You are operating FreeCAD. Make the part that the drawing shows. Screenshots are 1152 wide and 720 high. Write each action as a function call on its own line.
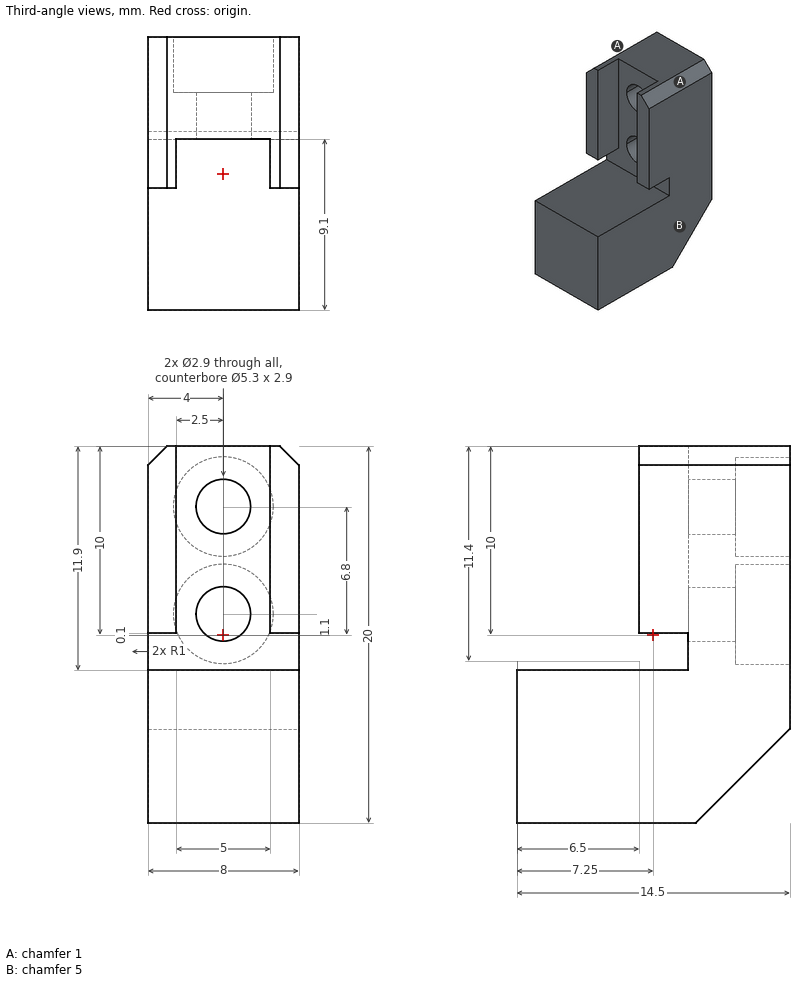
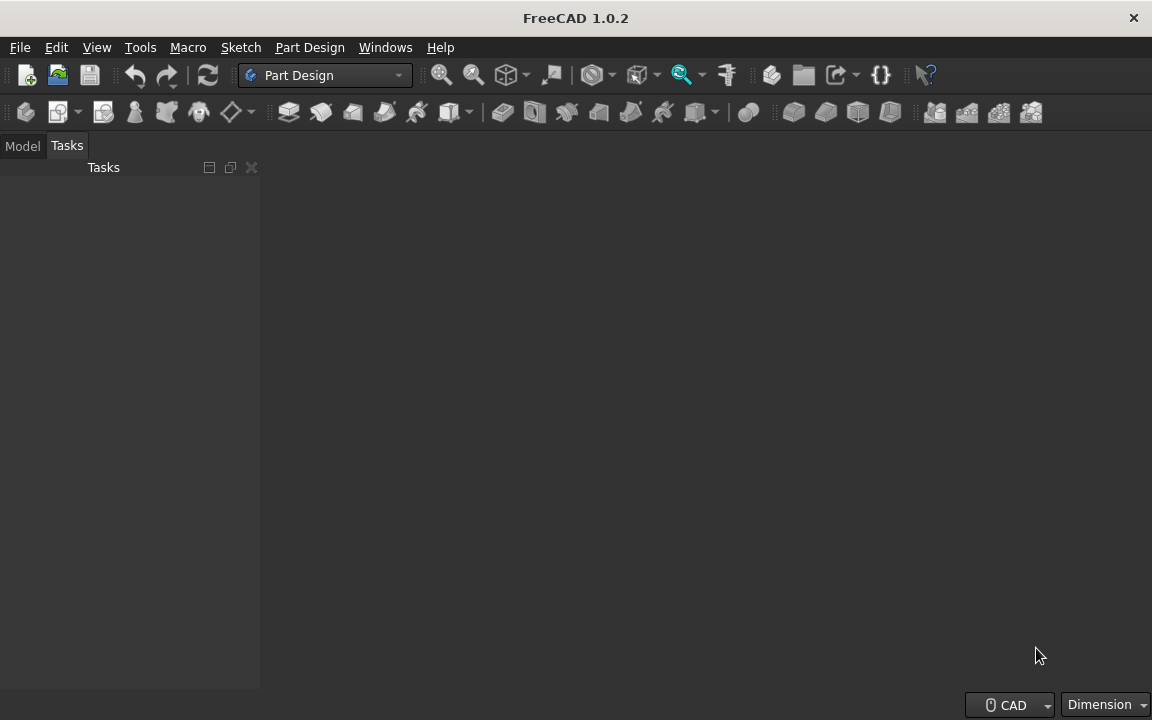
key(ctrl+n)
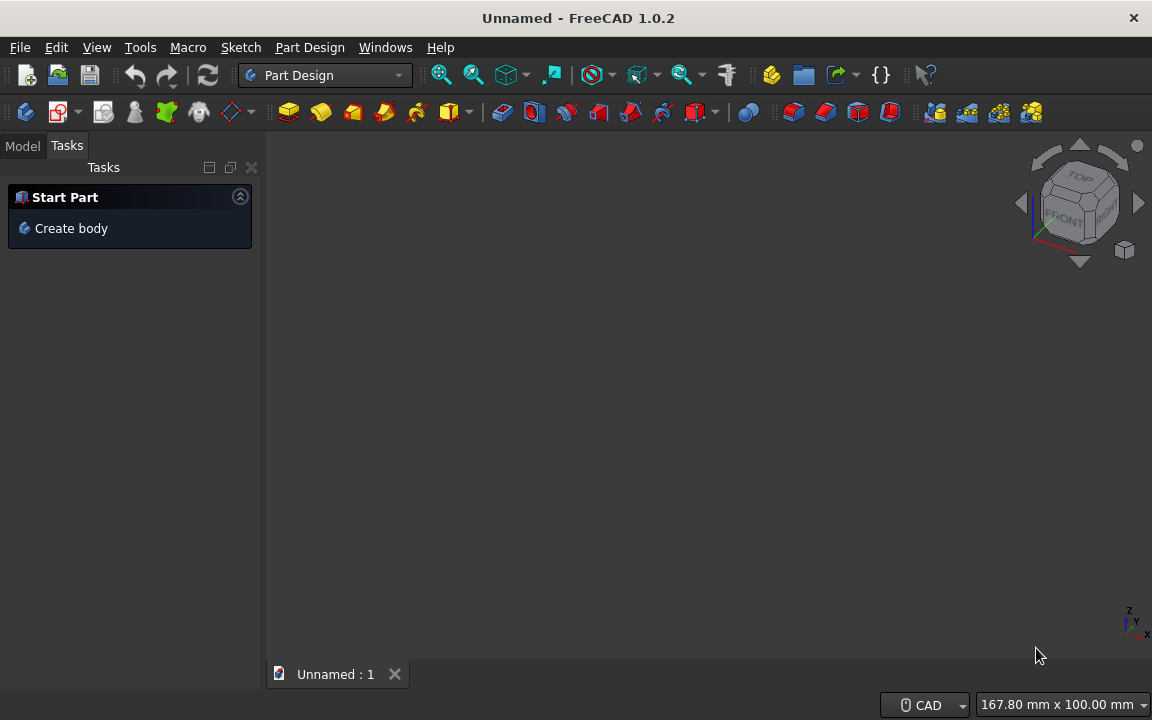
click(58, 112)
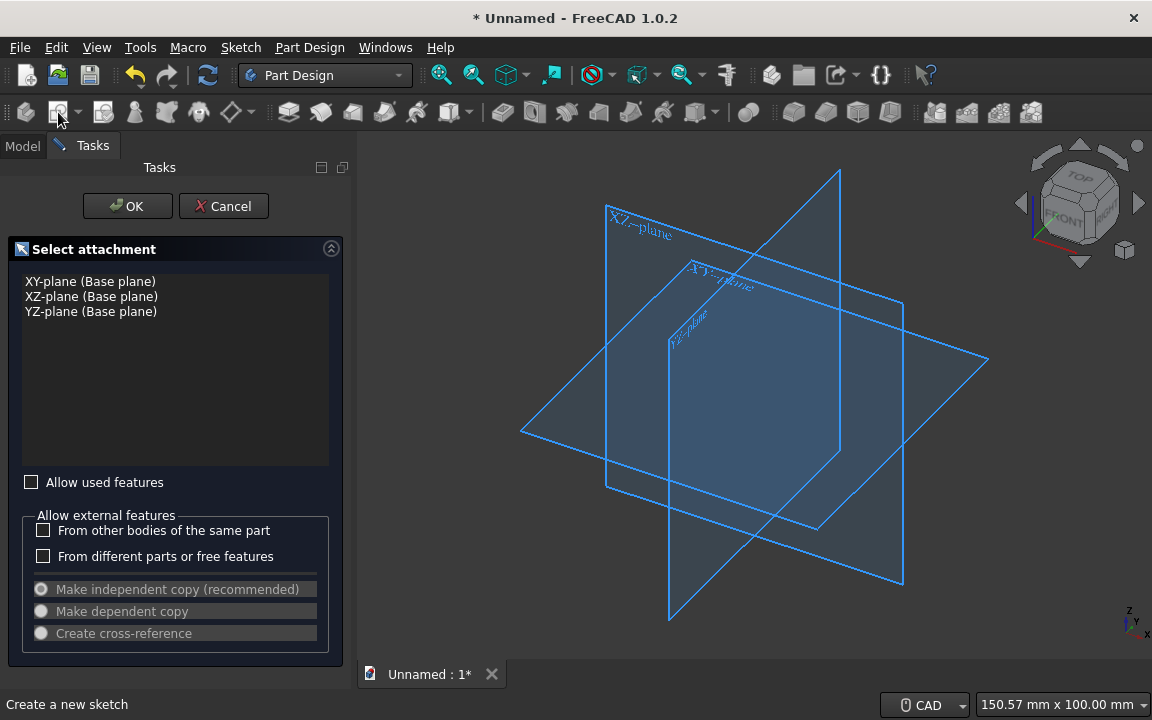
click(82, 296)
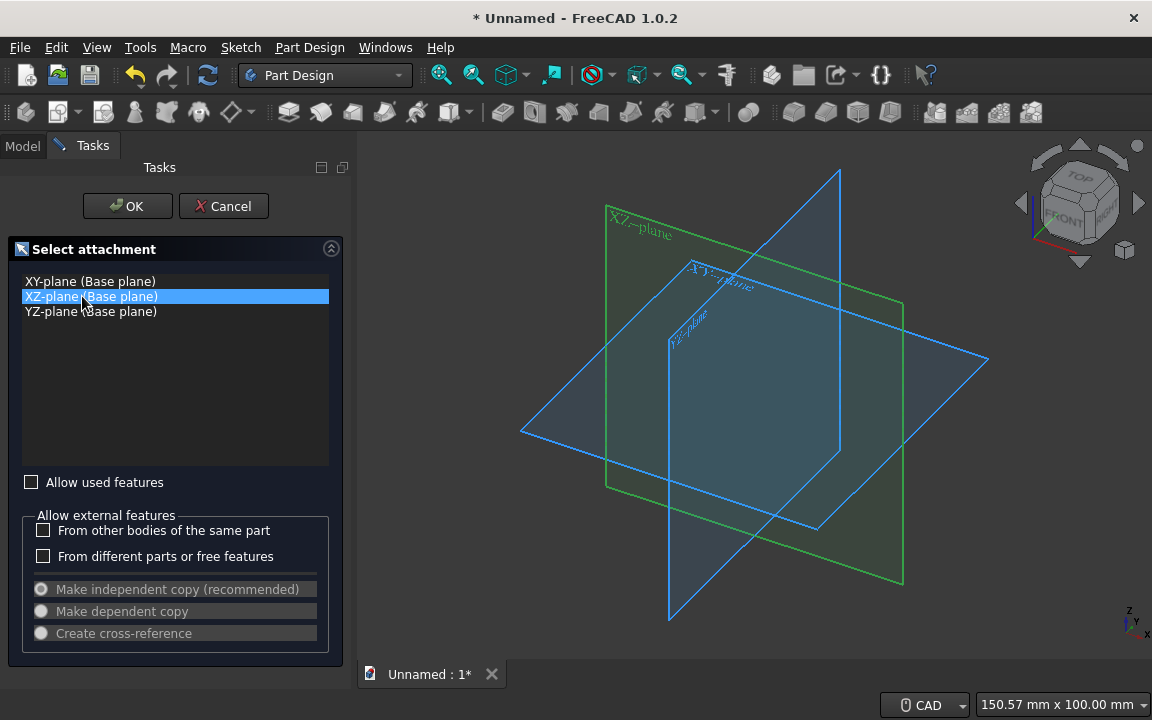
click(128, 206)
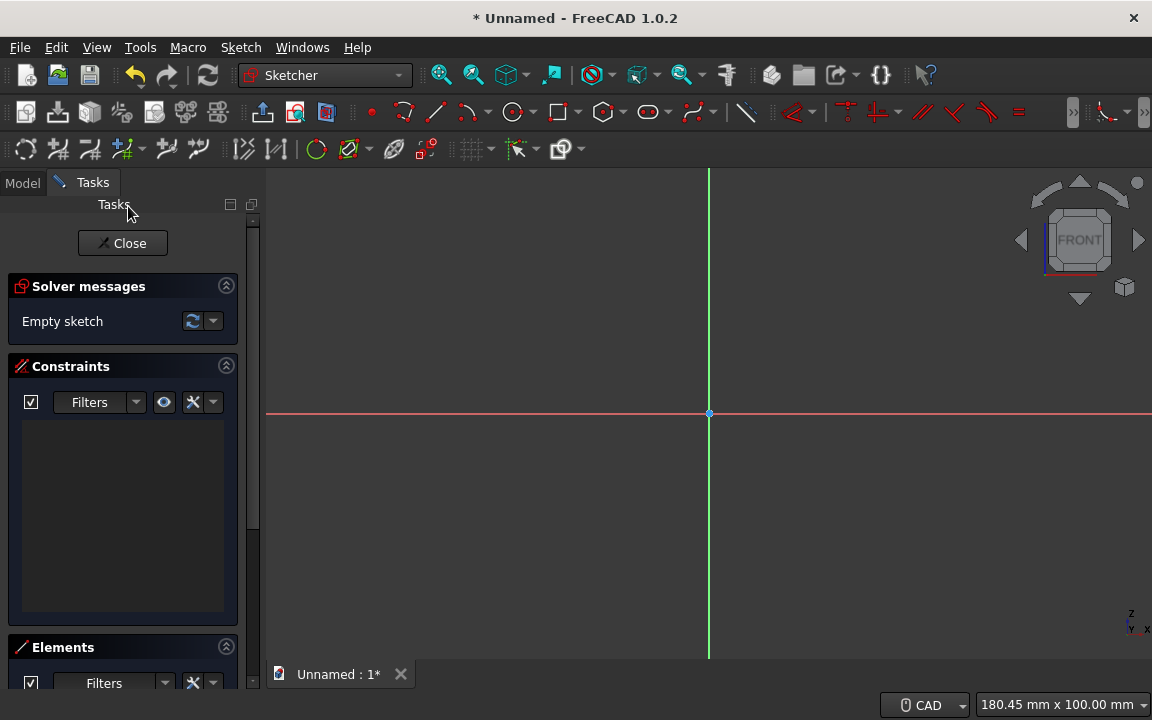
scroll(739, 414, up, 6)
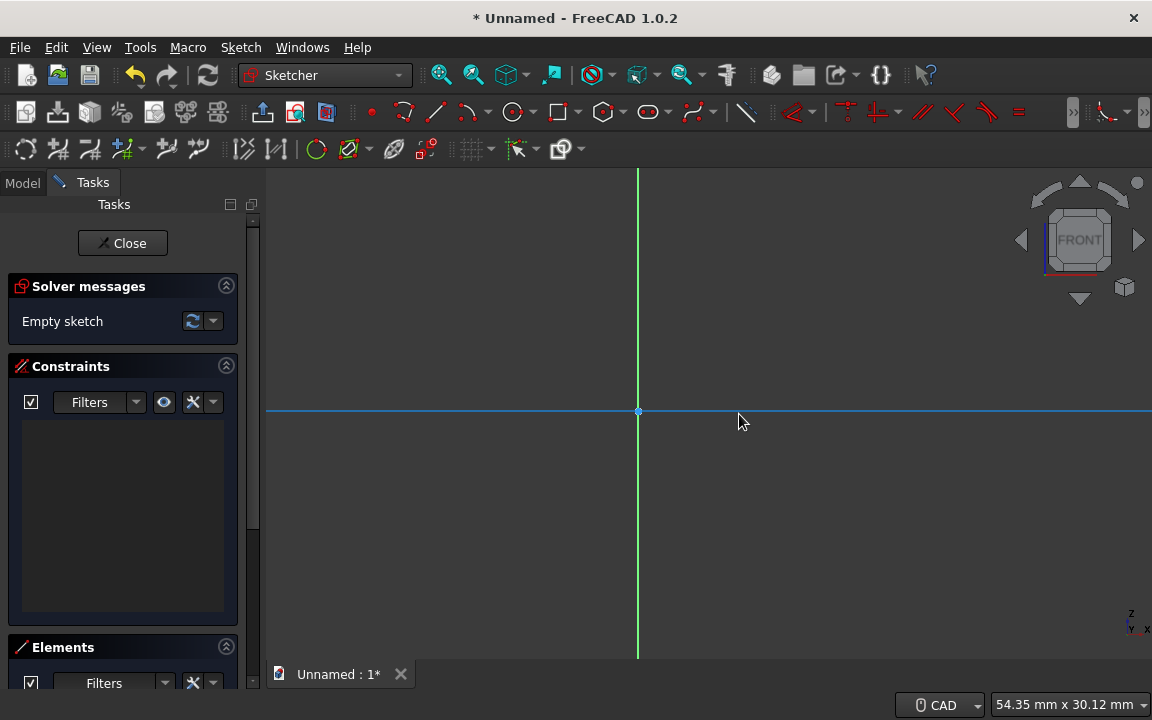
key(g)
key(v)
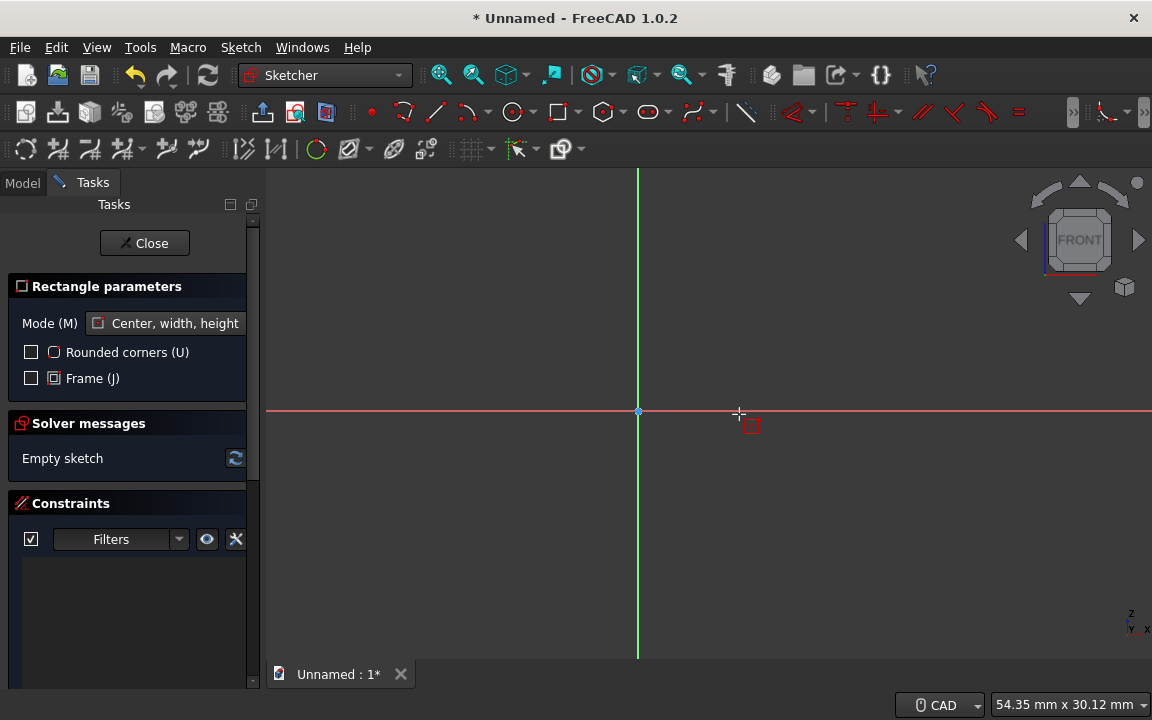
click(638, 411)
click(703, 248)
key(Escape)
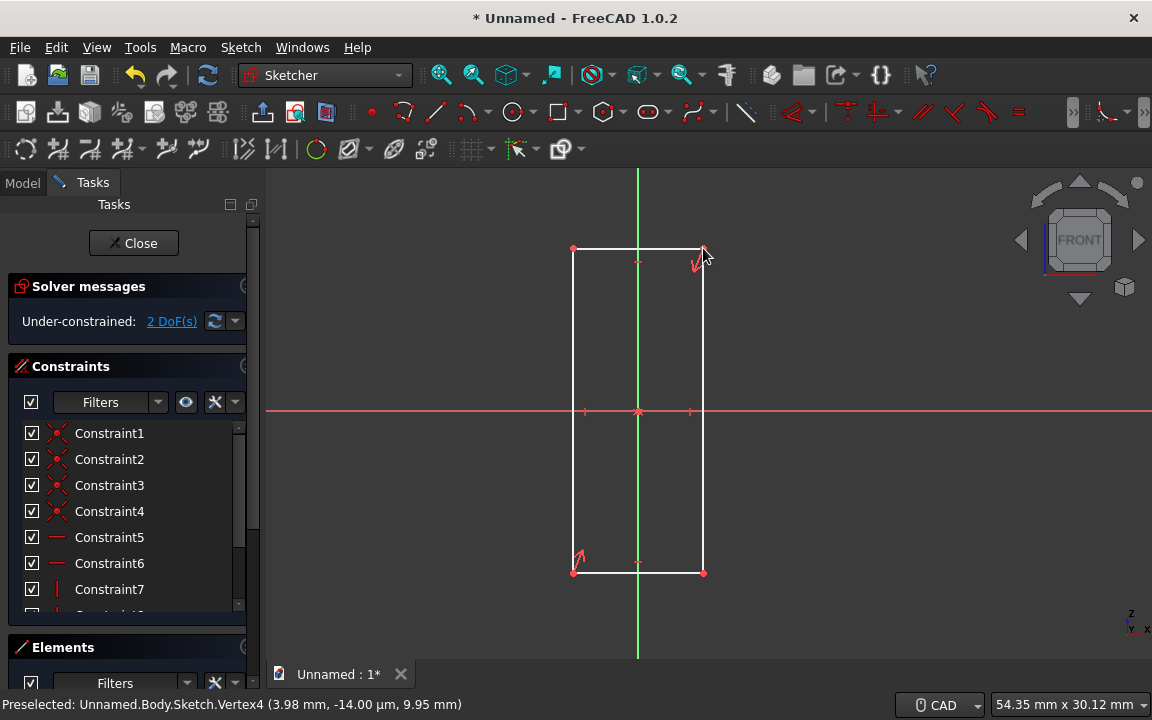
key(d)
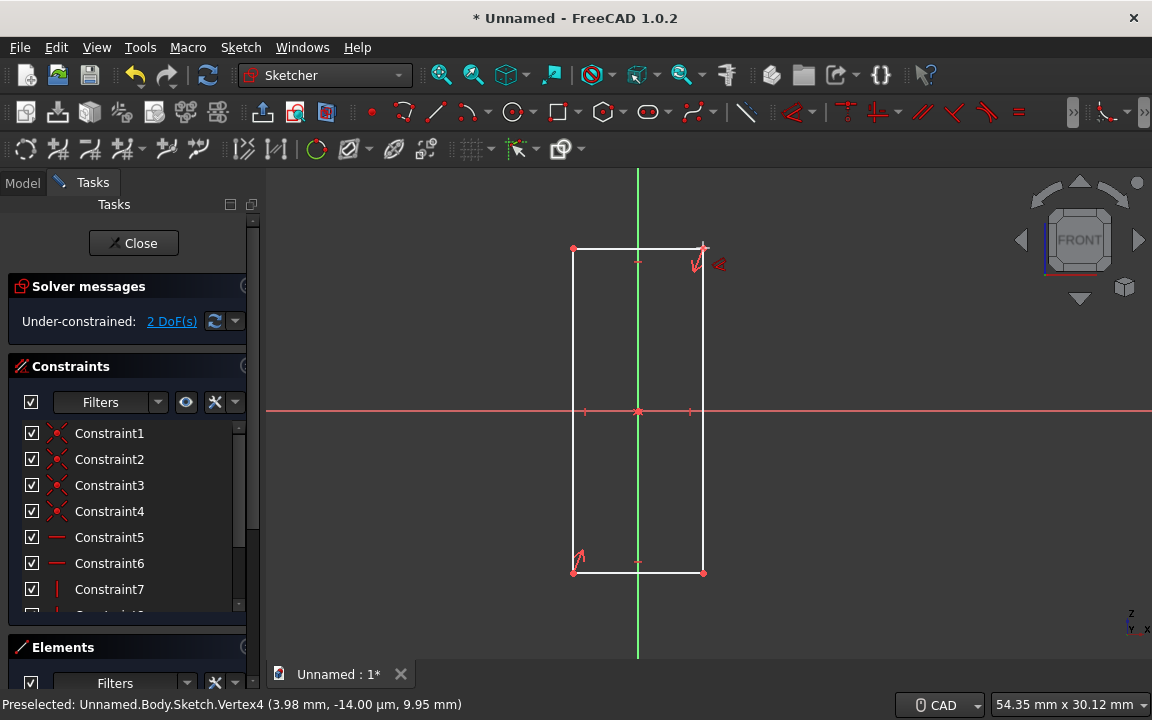
click(612, 573)
click(608, 607)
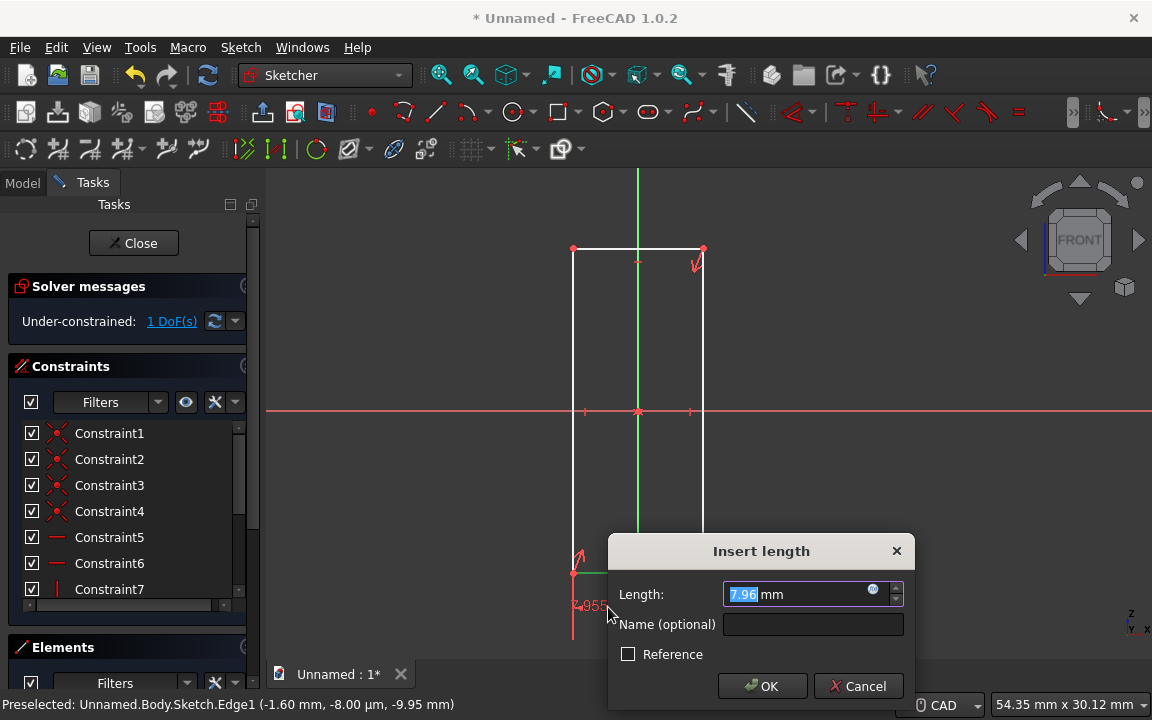
text(8)
key(Return)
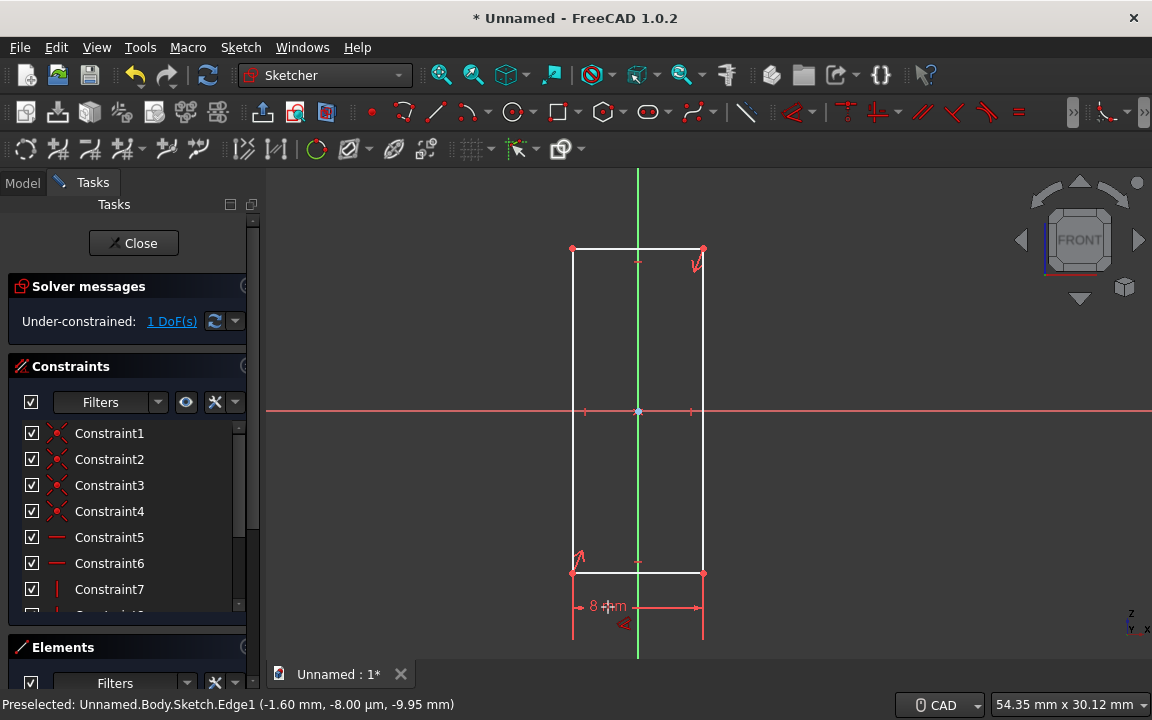
click(703, 476)
click(737, 337)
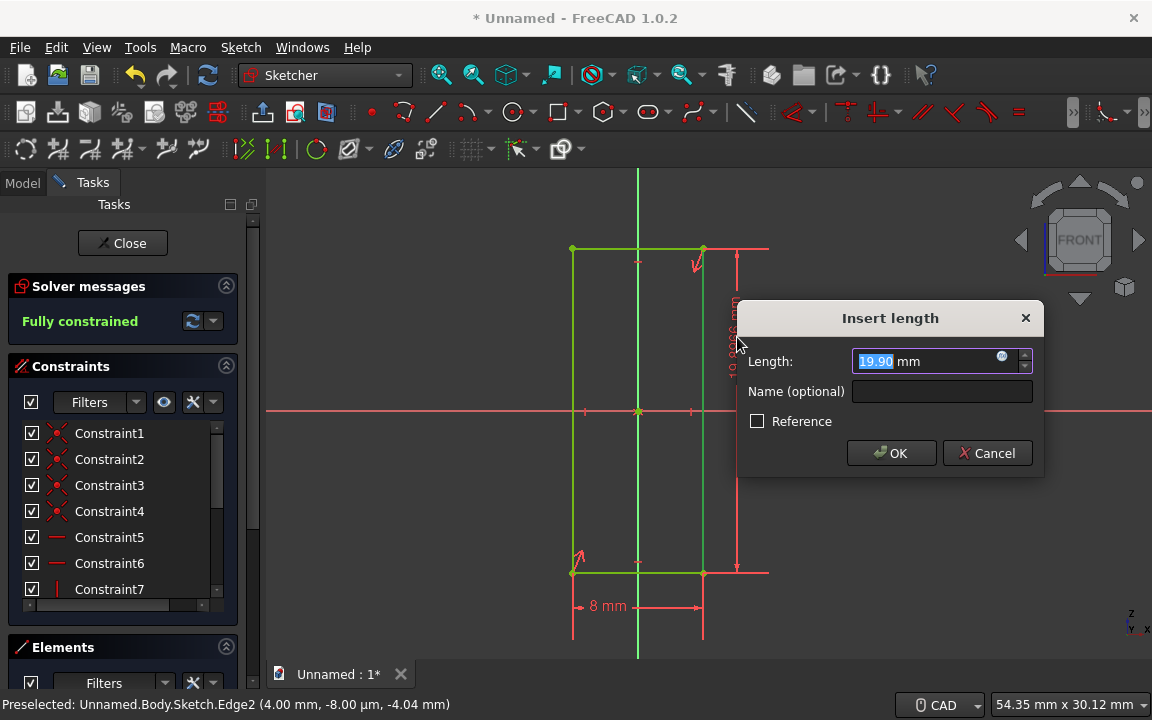
text(20)
key(Return)
key(Escape)